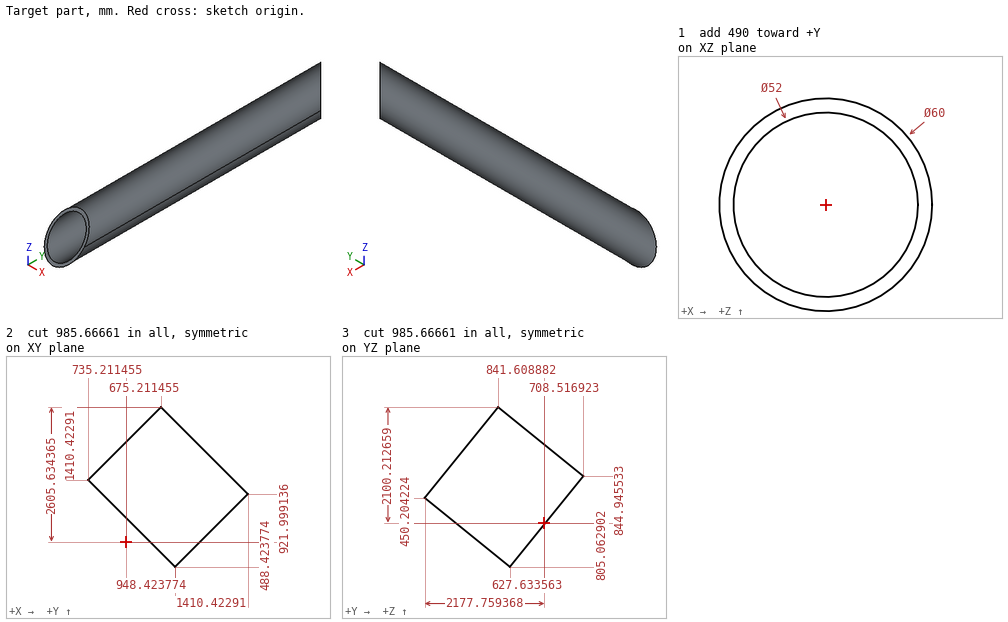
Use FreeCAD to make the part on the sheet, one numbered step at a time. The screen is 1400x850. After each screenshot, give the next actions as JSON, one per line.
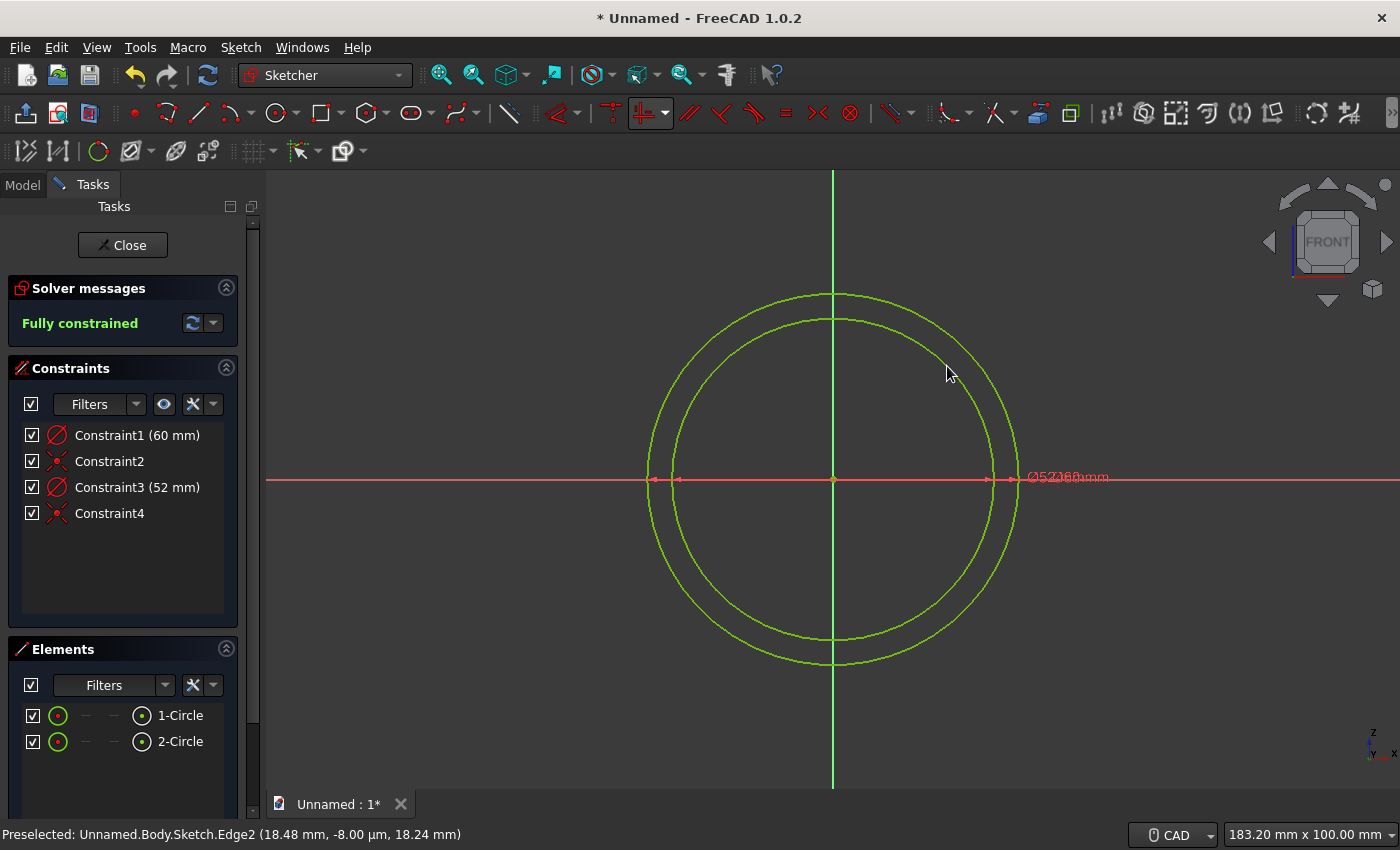
{"action": "left_click", "coordinate": [123, 245]}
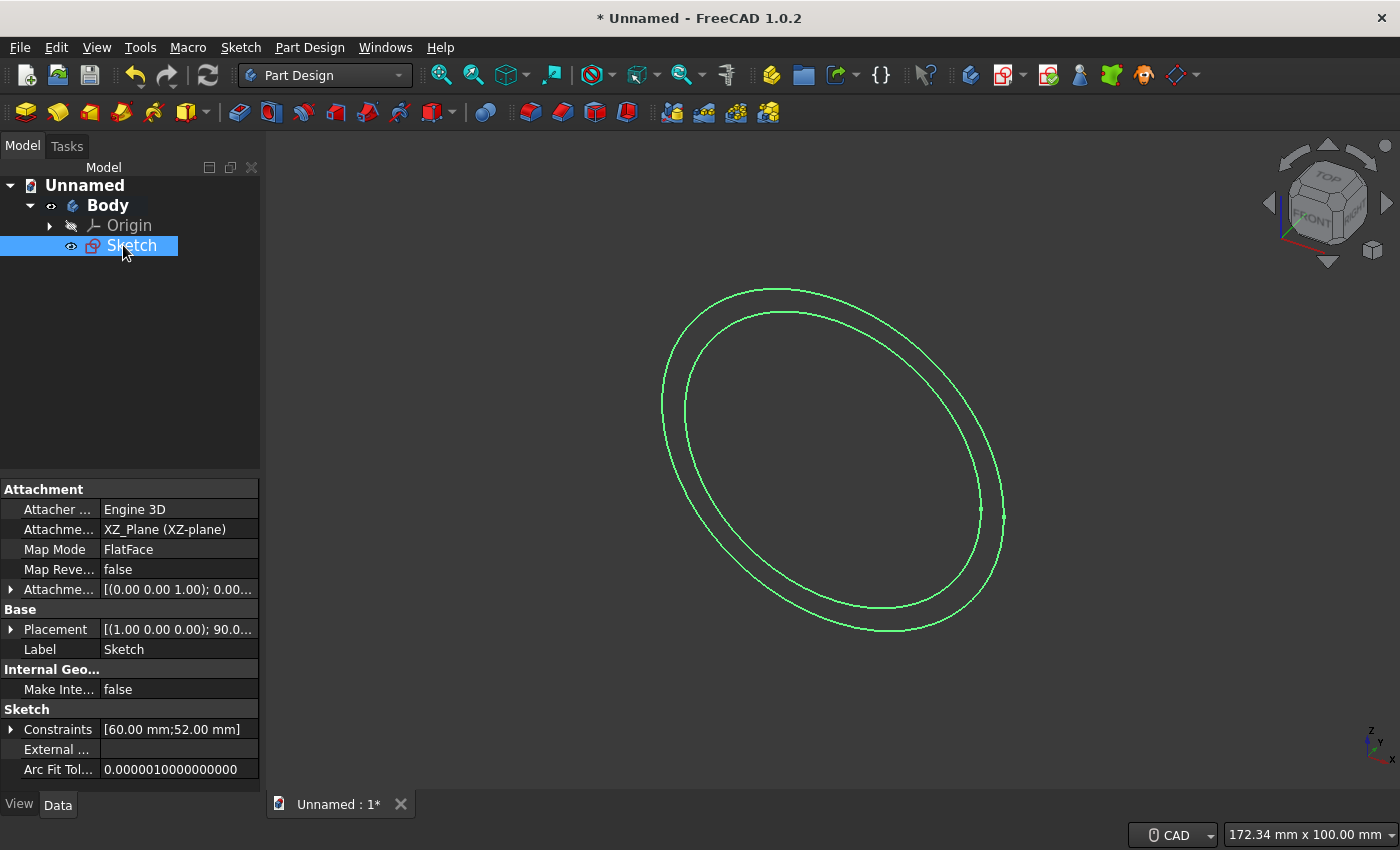
{"action": "left_click", "coordinate": [26, 112]}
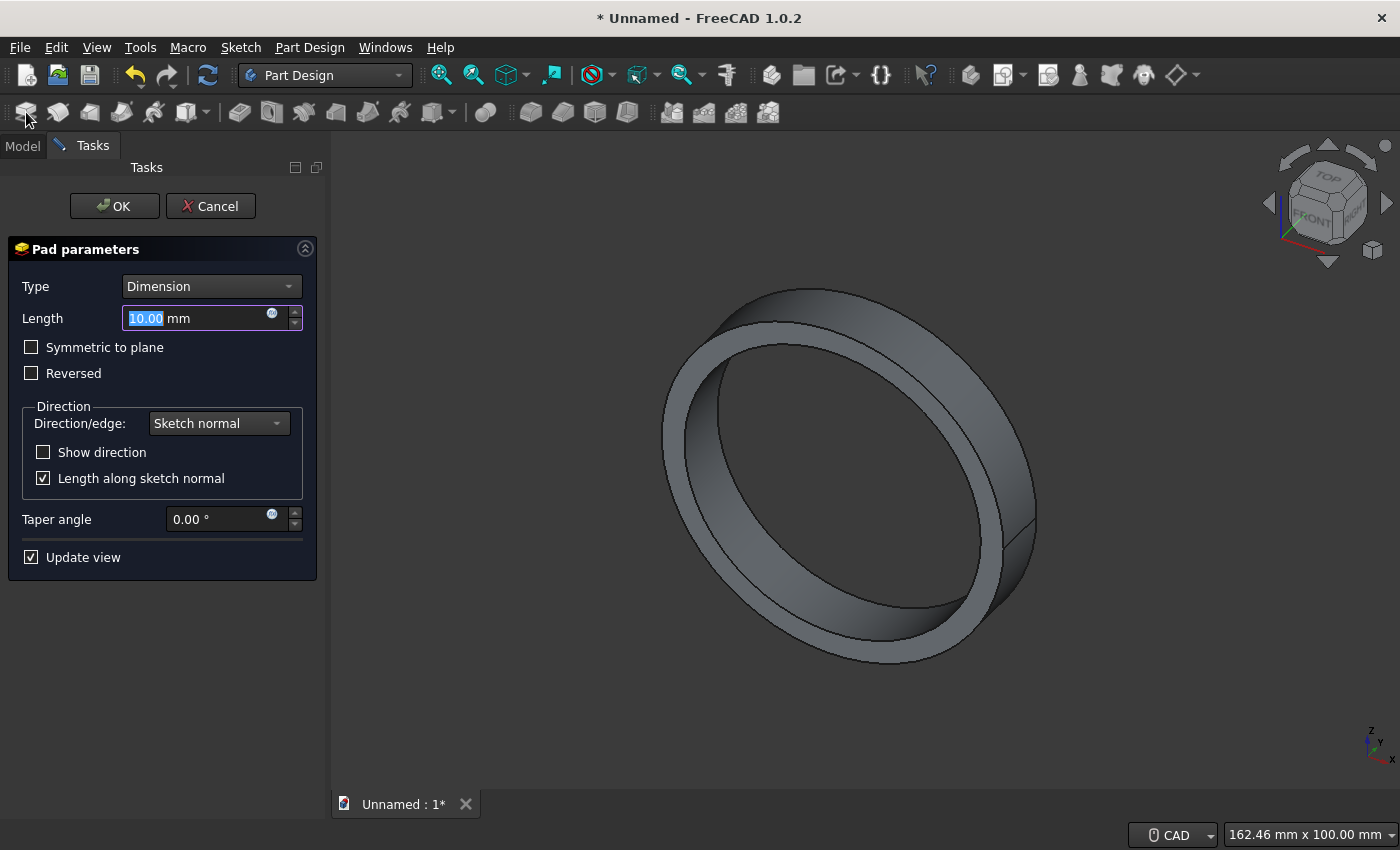
{"action": "type", "text": "490"}
{"action": "key", "text": "Tab"}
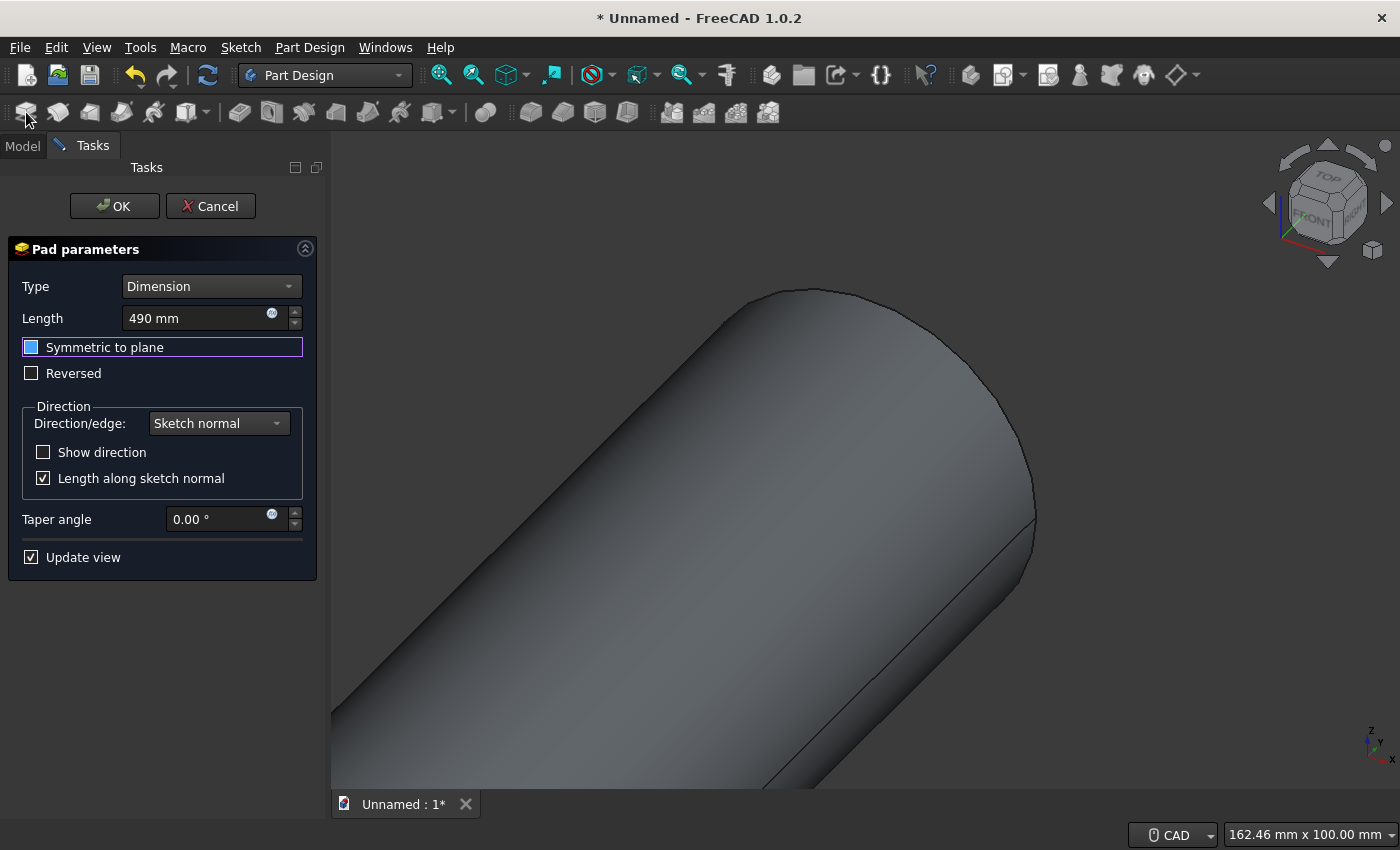
{"action": "left_click", "coordinate": [30, 373]}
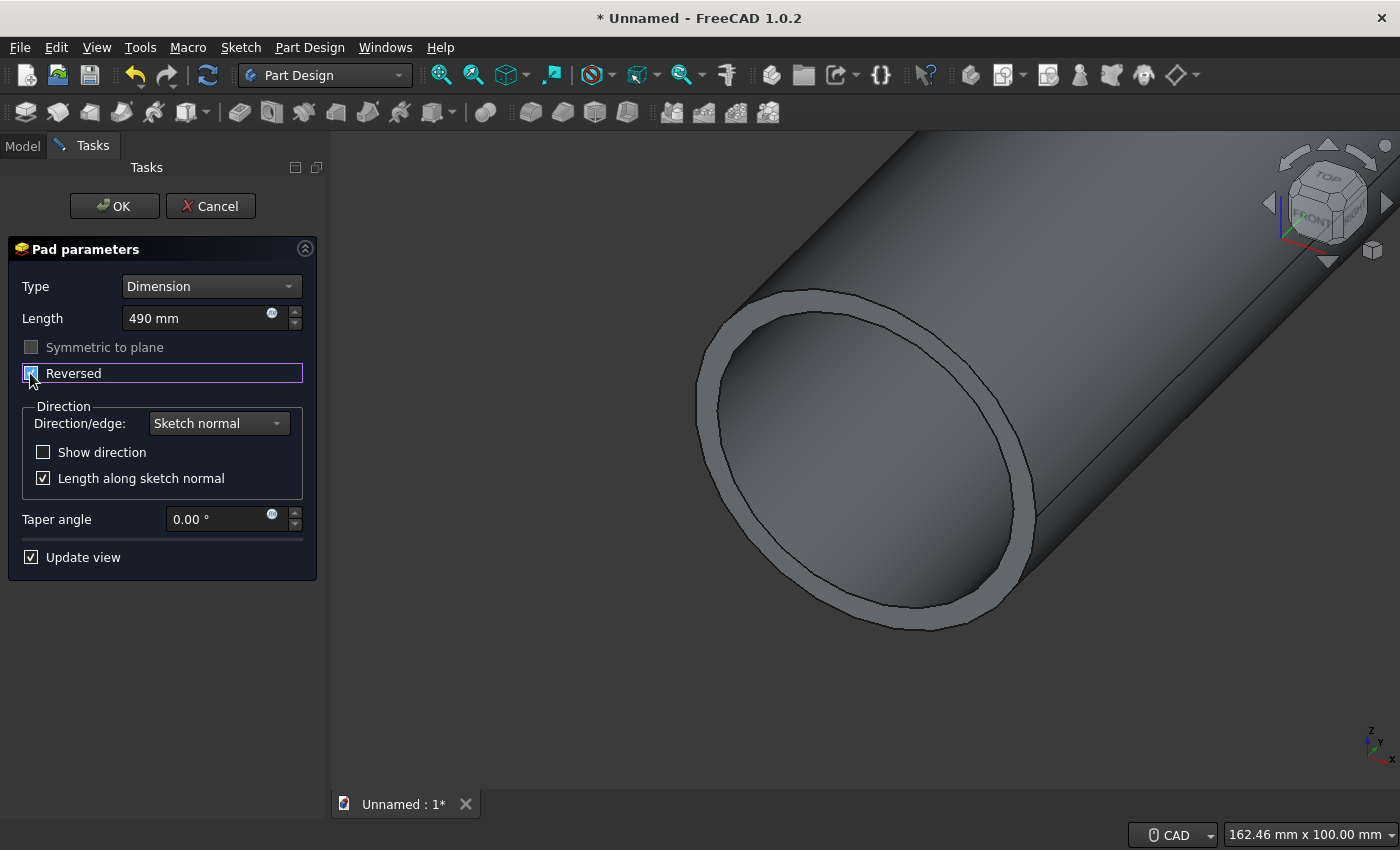
{"action": "left_click", "coordinate": [115, 206]}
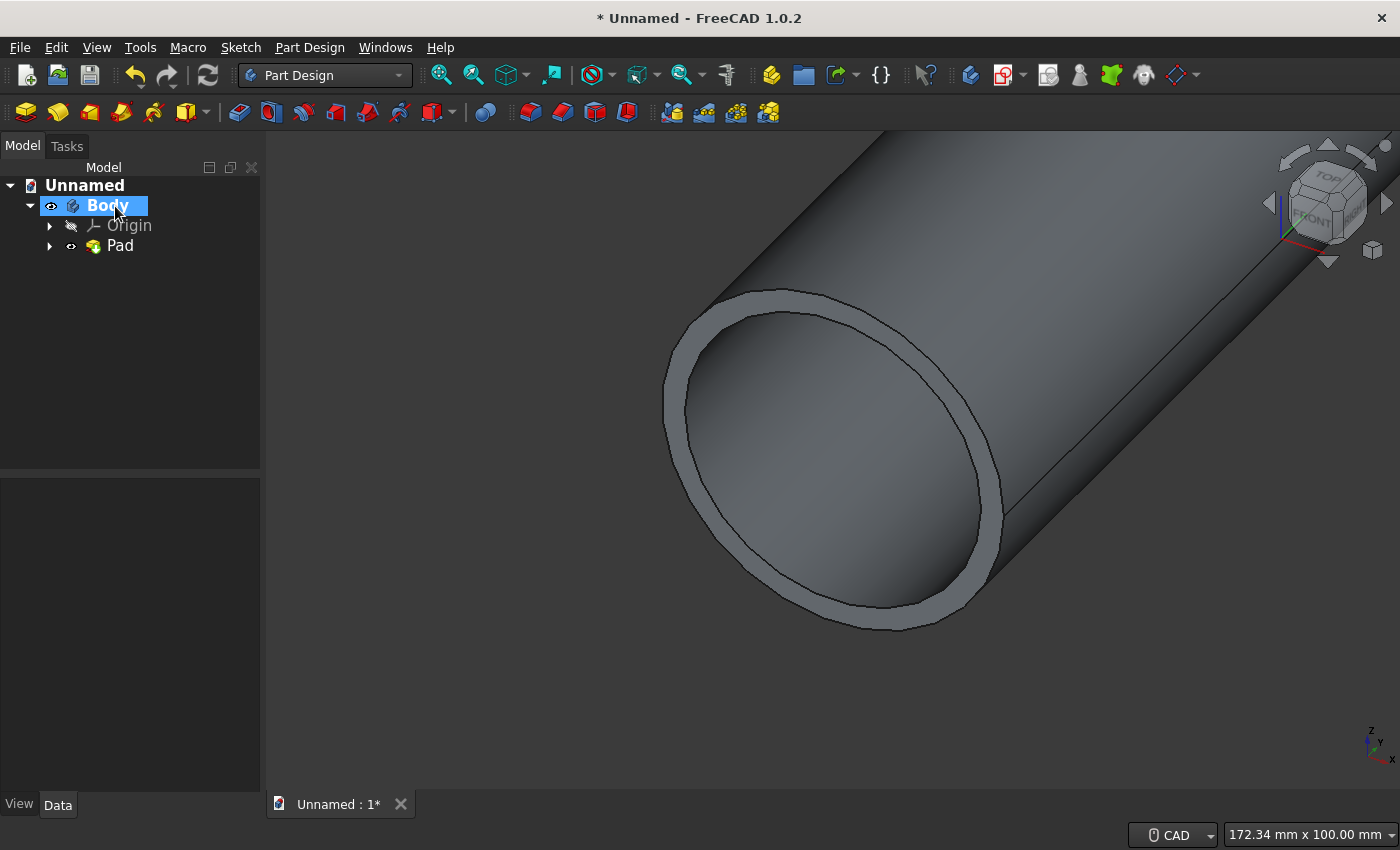
{"action": "key", "text": "v f"}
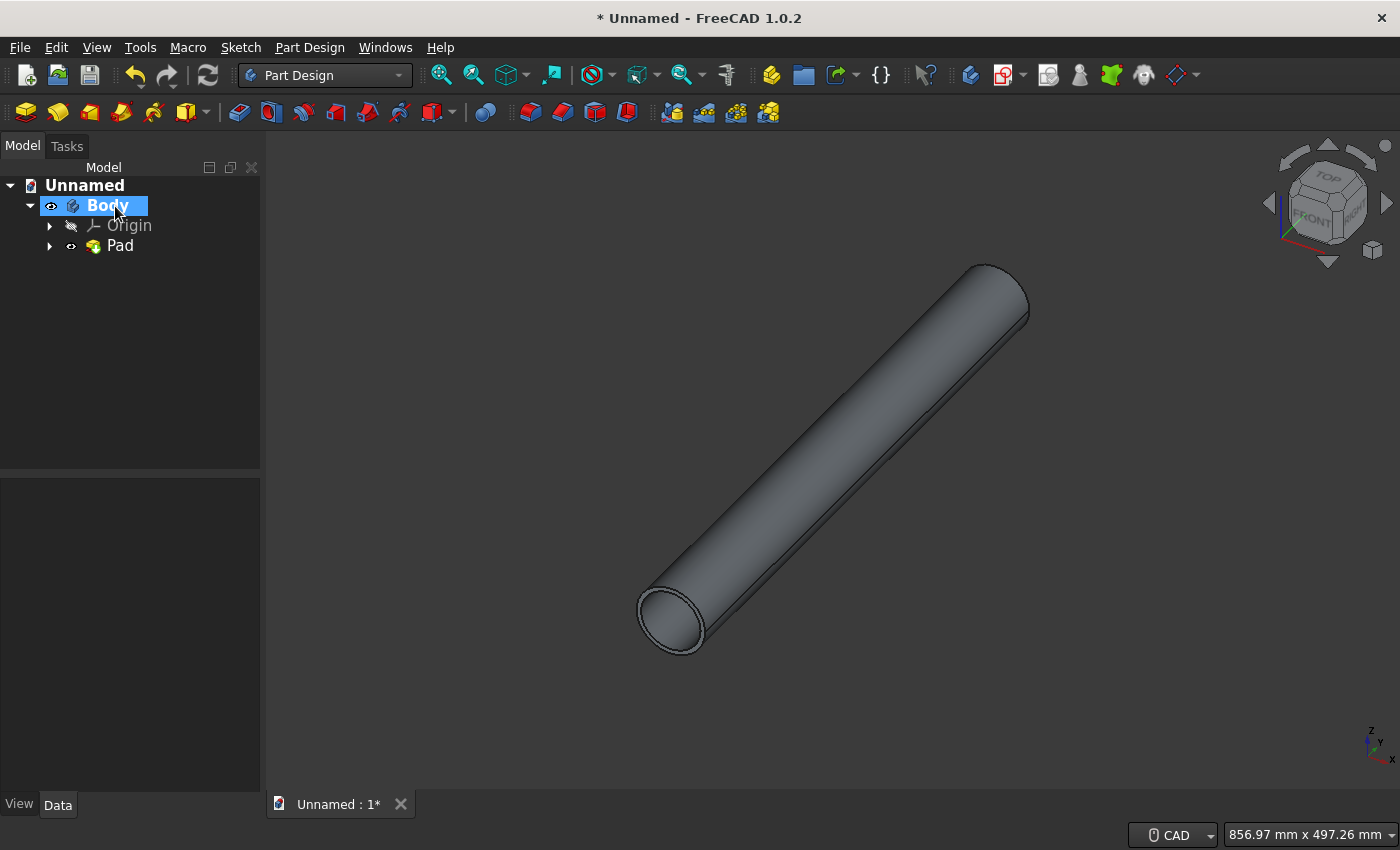
{"action": "left_click", "coordinate": [1004, 76]}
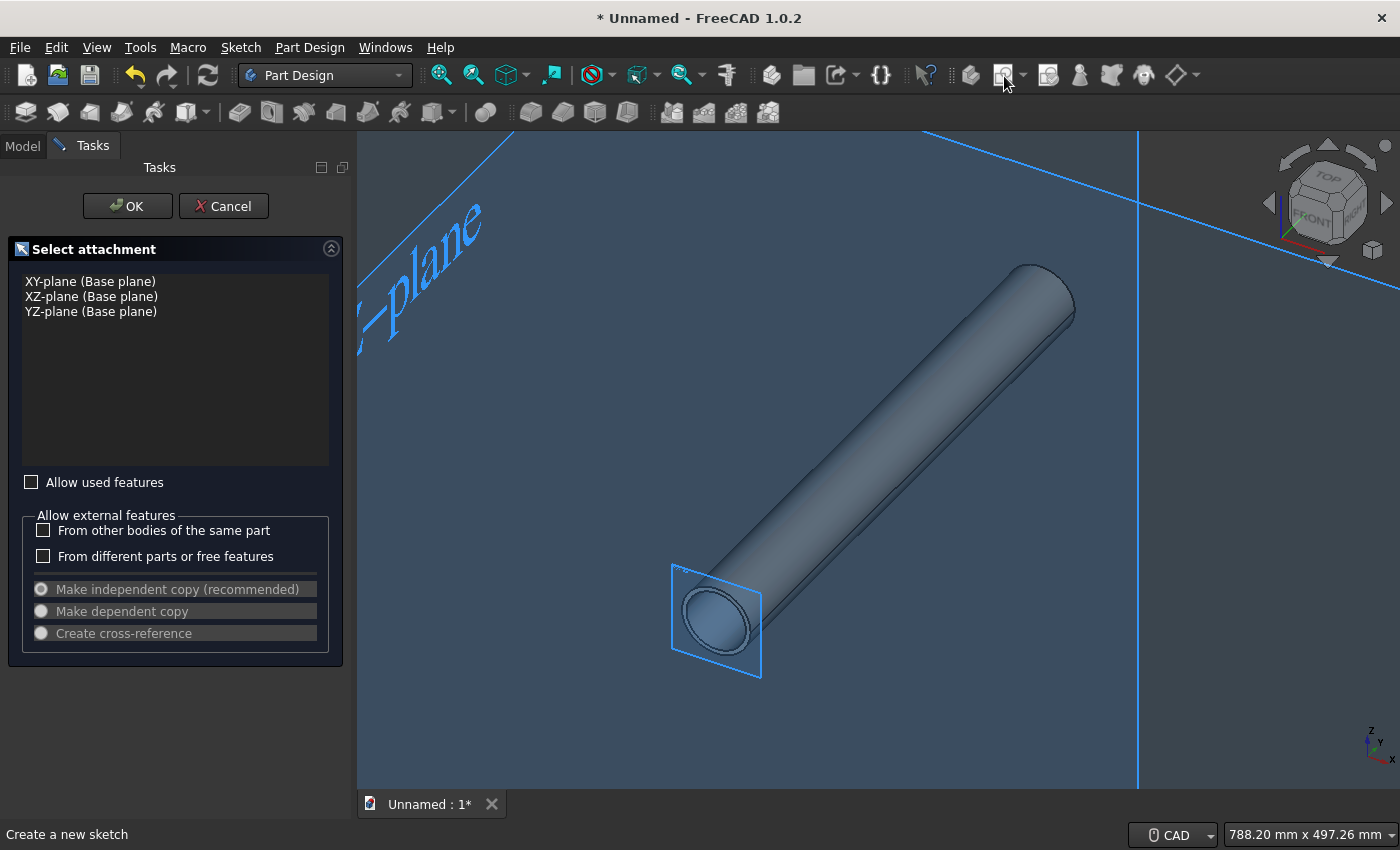
{"action": "left_click", "coordinate": [82, 282]}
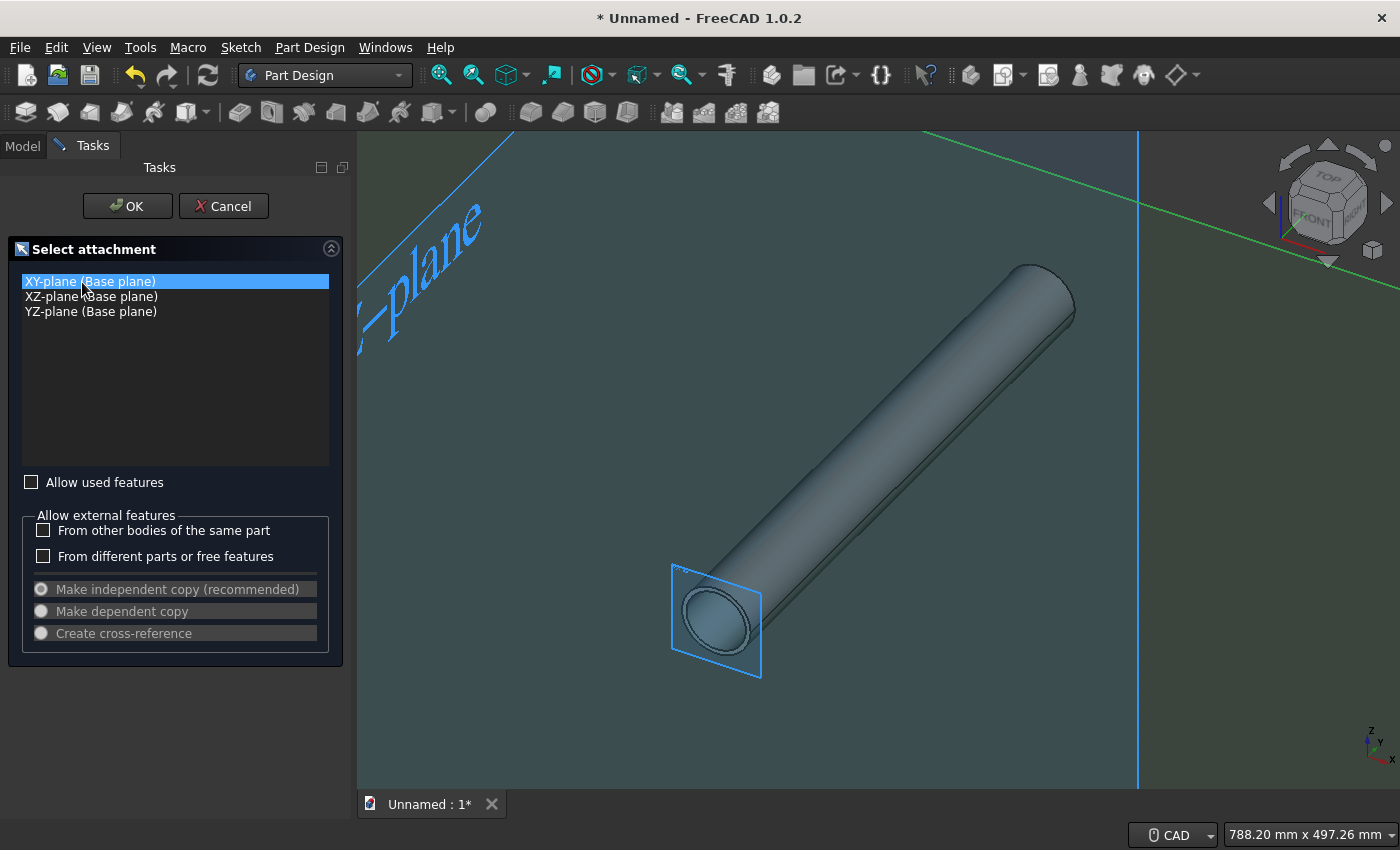
{"action": "left_click", "coordinate": [128, 206]}